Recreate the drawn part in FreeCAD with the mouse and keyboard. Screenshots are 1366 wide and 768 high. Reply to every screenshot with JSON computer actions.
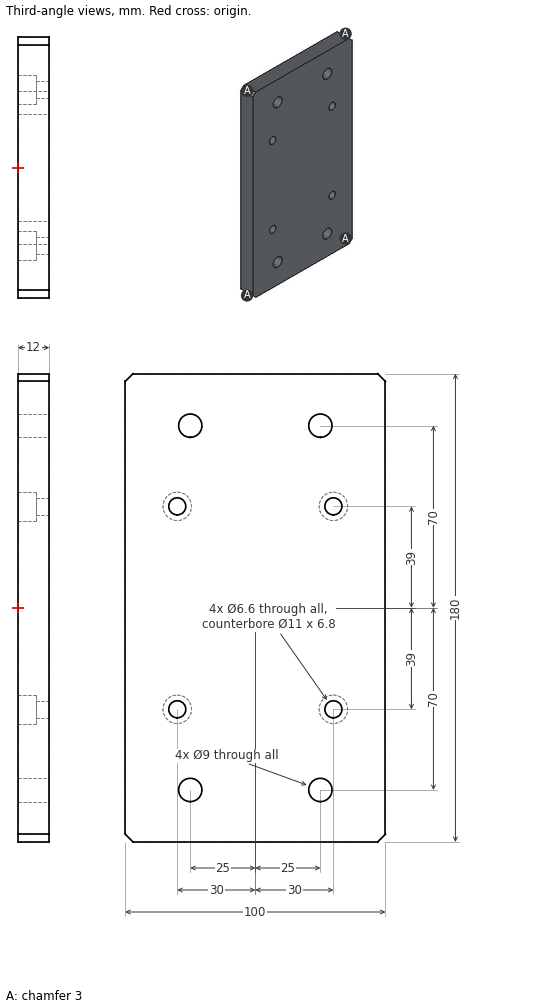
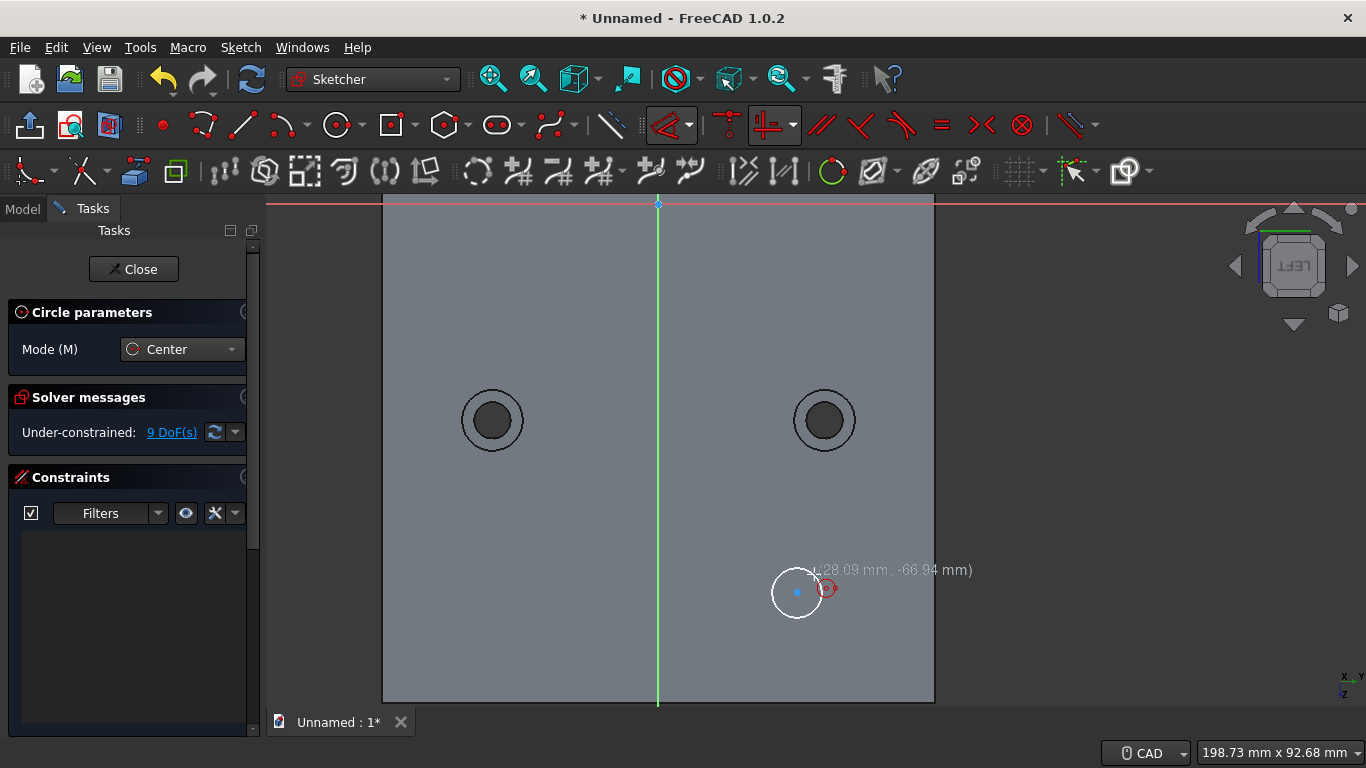
{"action": "left_click", "coordinate": [520, 592]}
{"action": "left_click", "coordinate": [538, 574]}
{"action": "key", "text": "Escape"}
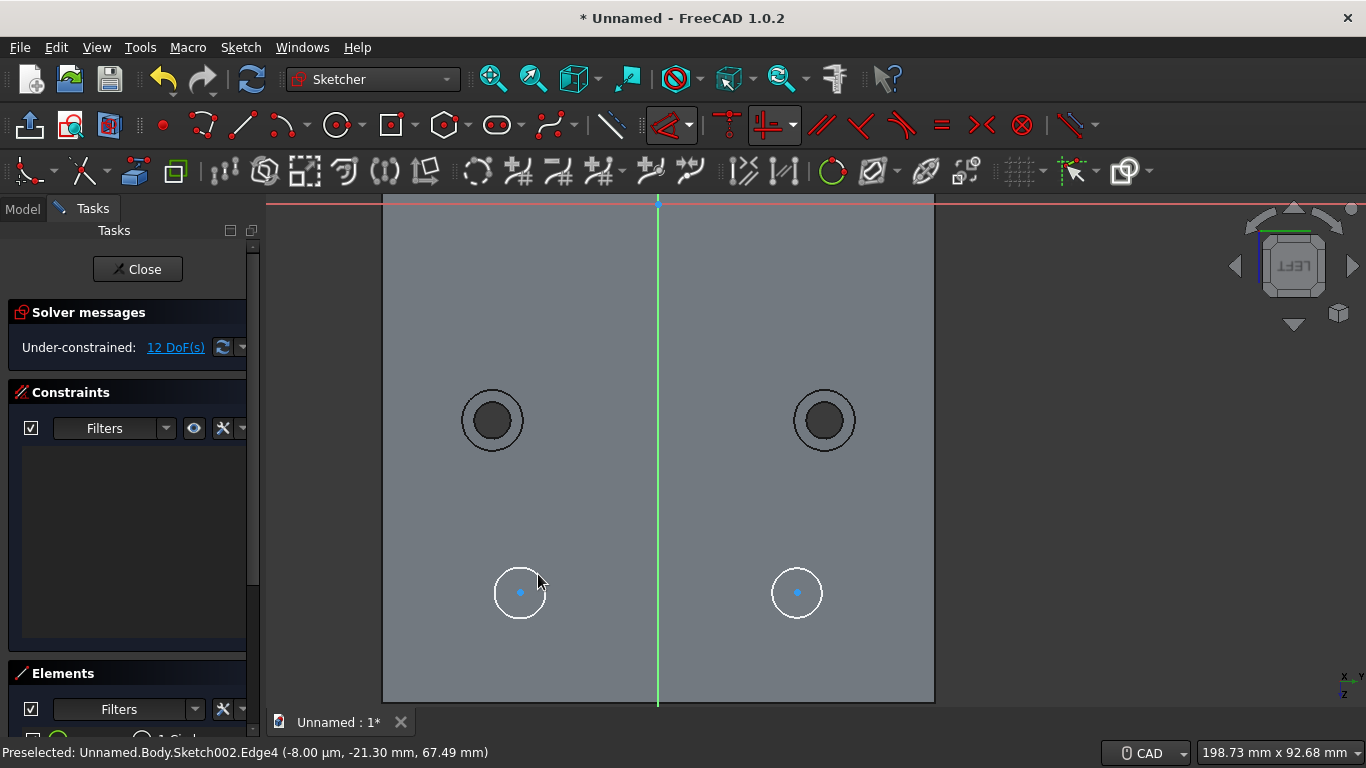
{"action": "scroll", "coordinate": [799, 594], "scroll_direction": "down", "scroll_amount": 5}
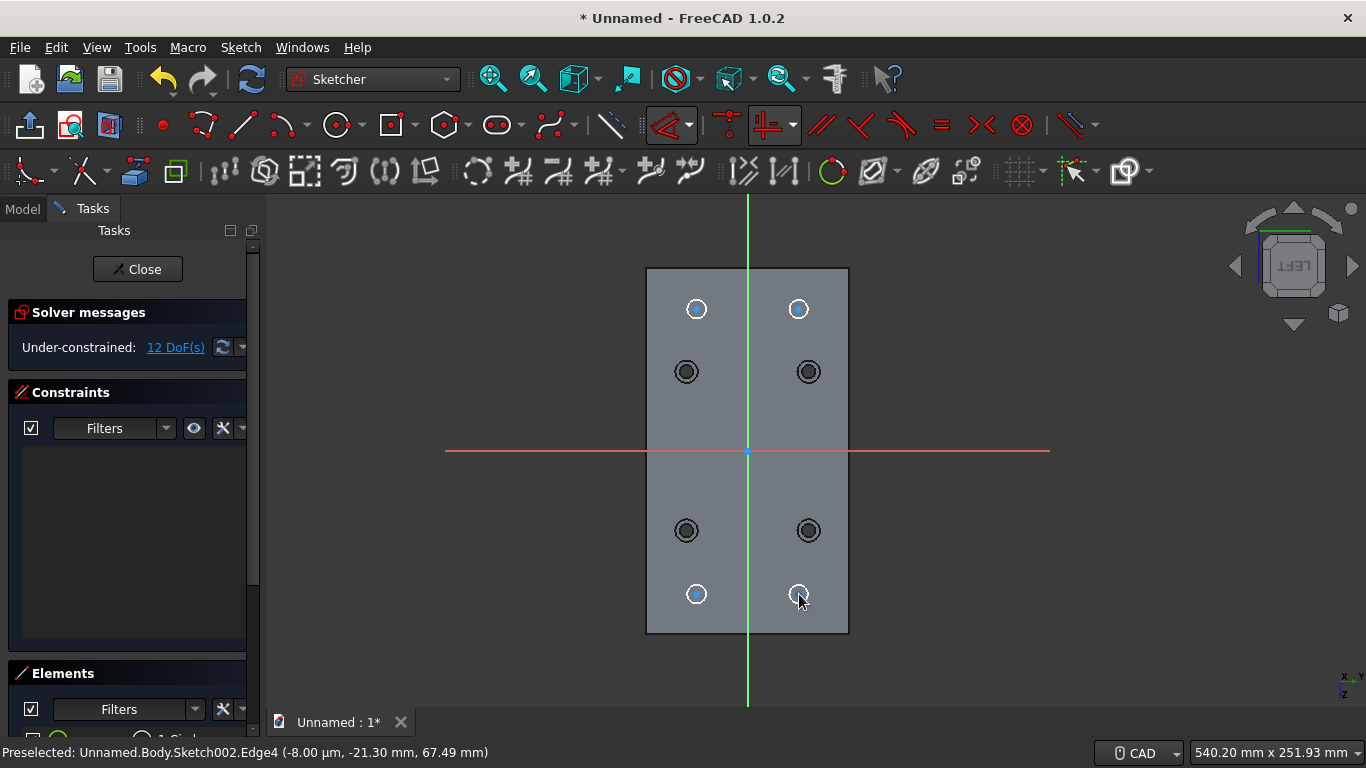
{"action": "scroll", "coordinate": [805, 303], "scroll_direction": "up", "scroll_amount": 3}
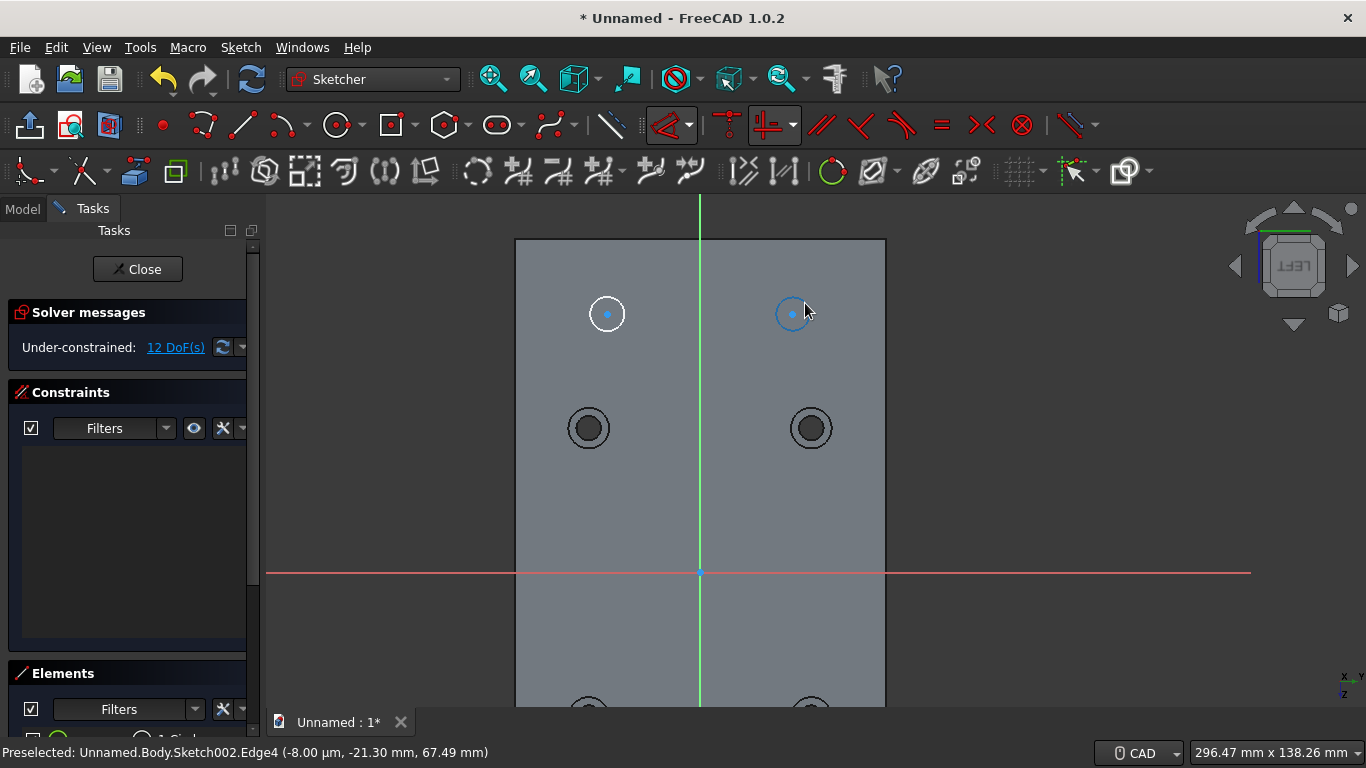
{"action": "left_click", "coordinate": [805, 302]}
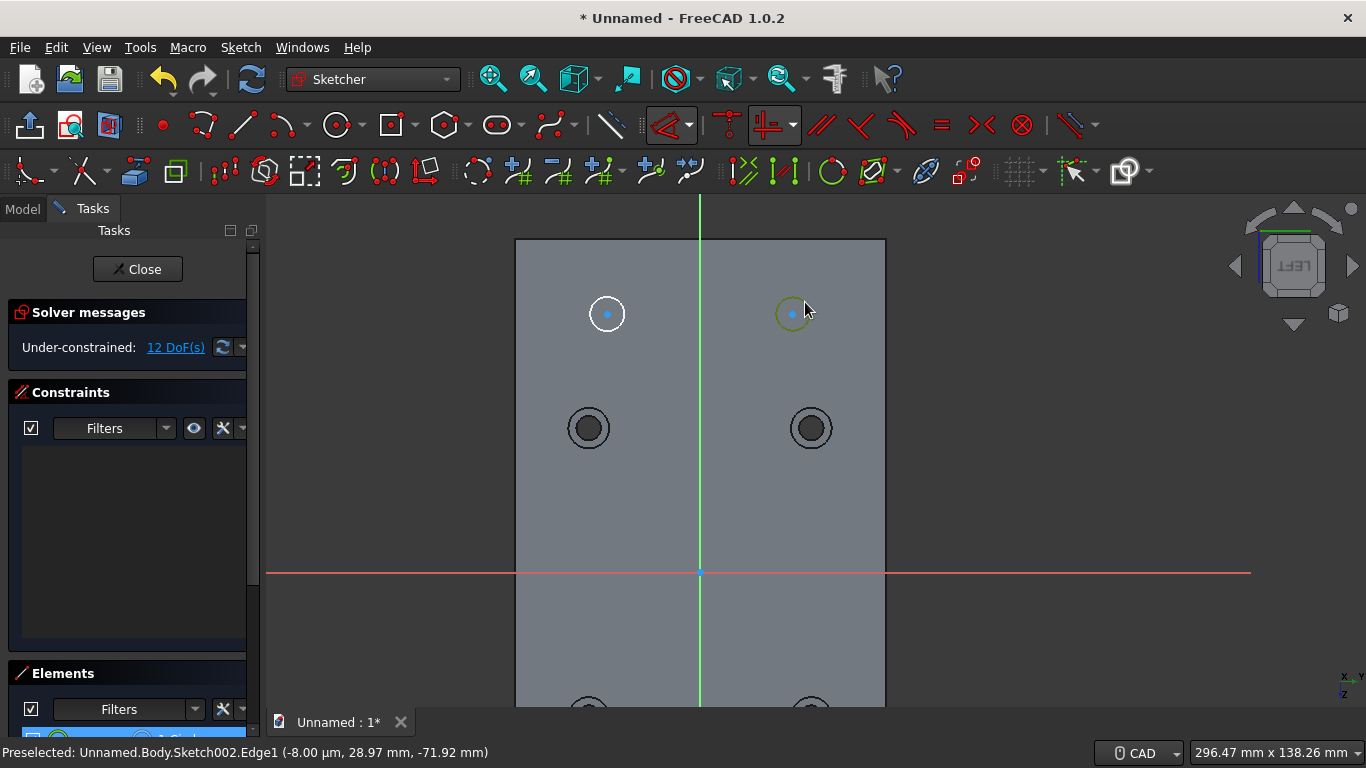
{"action": "left_click", "coordinate": [619, 302]}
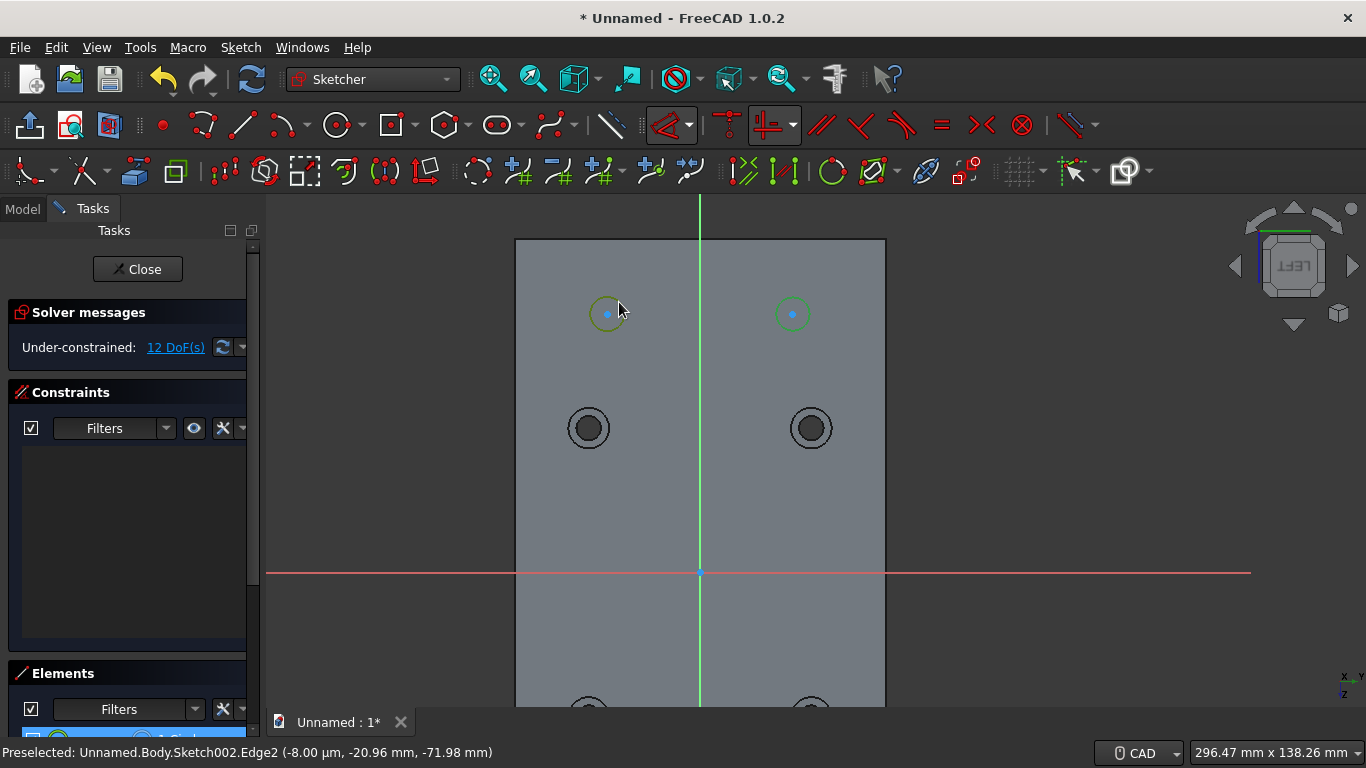
{"action": "scroll", "coordinate": [805, 302], "scroll_direction": "down", "scroll_amount": 3}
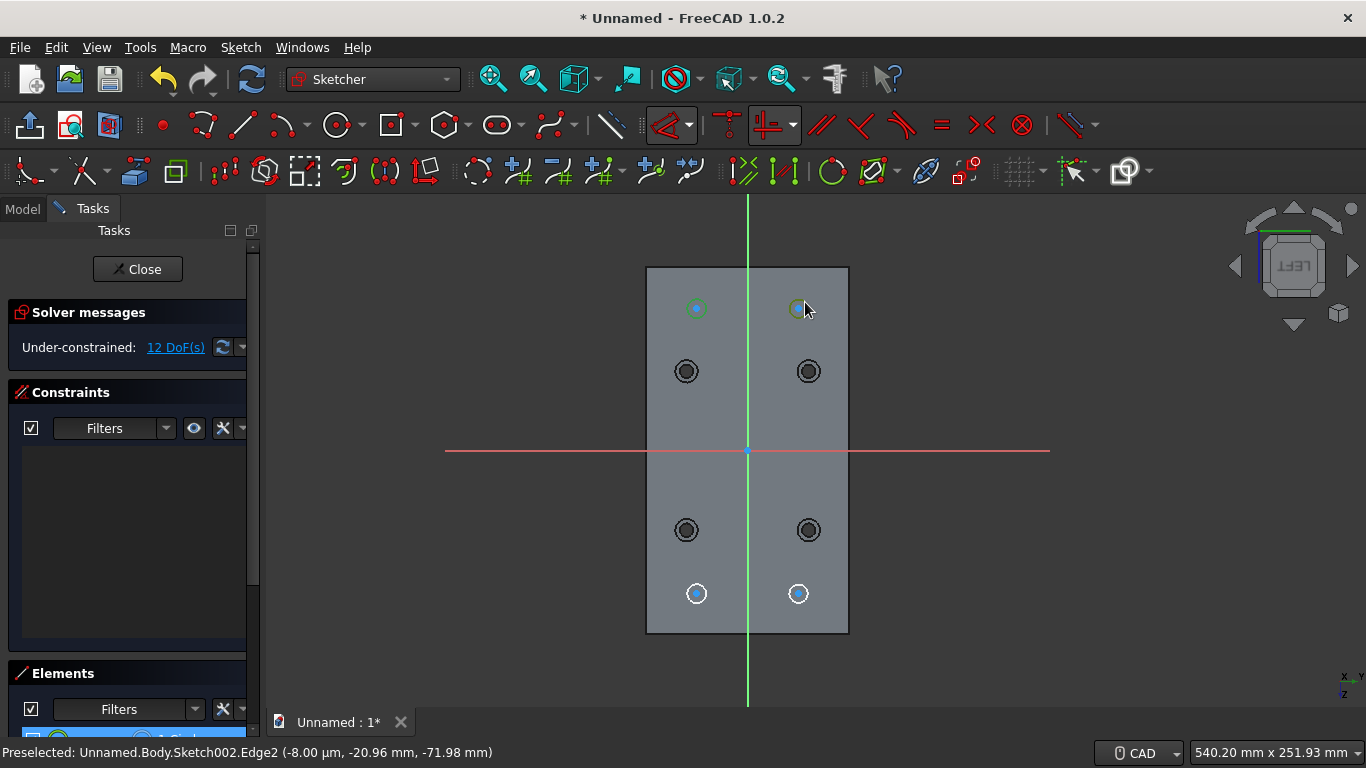
{"action": "scroll", "coordinate": [805, 587], "scroll_direction": "up", "scroll_amount": 3}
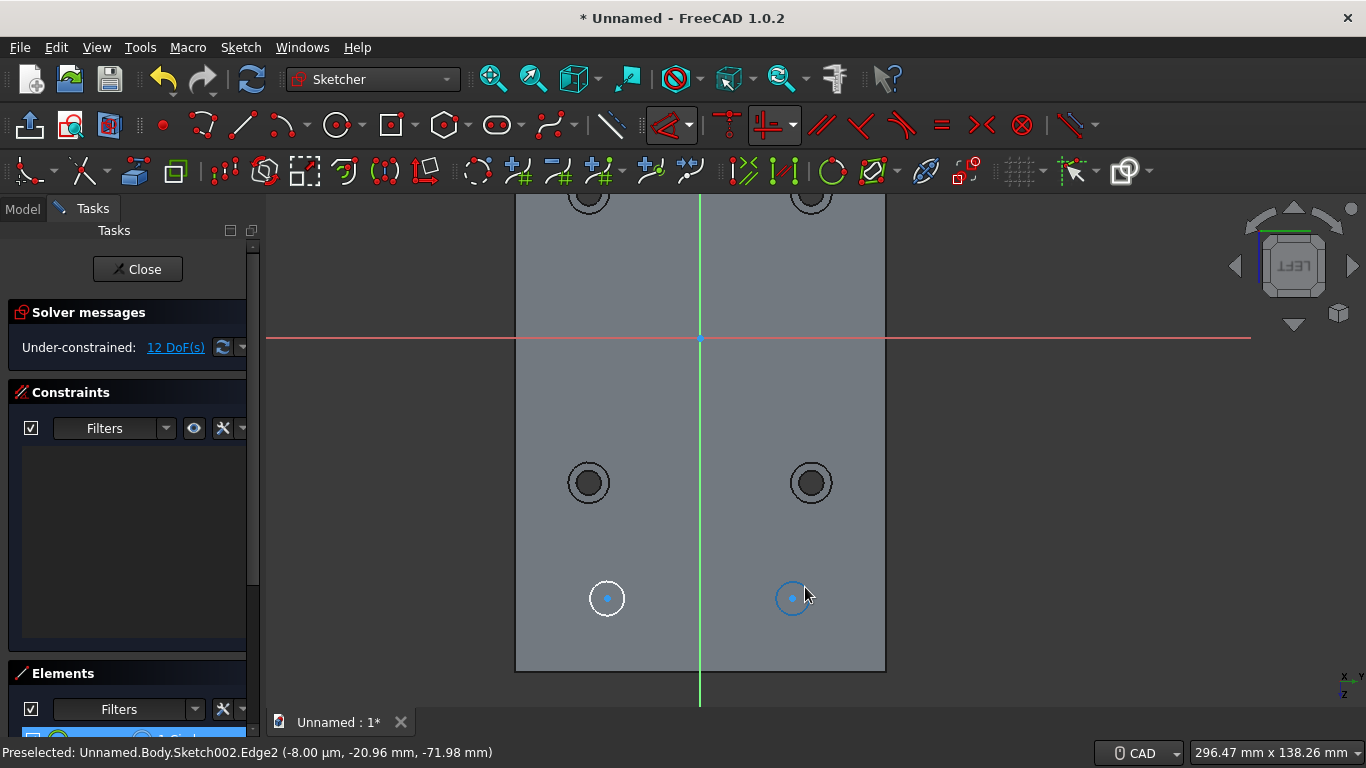
{"action": "left_click", "coordinate": [805, 587]}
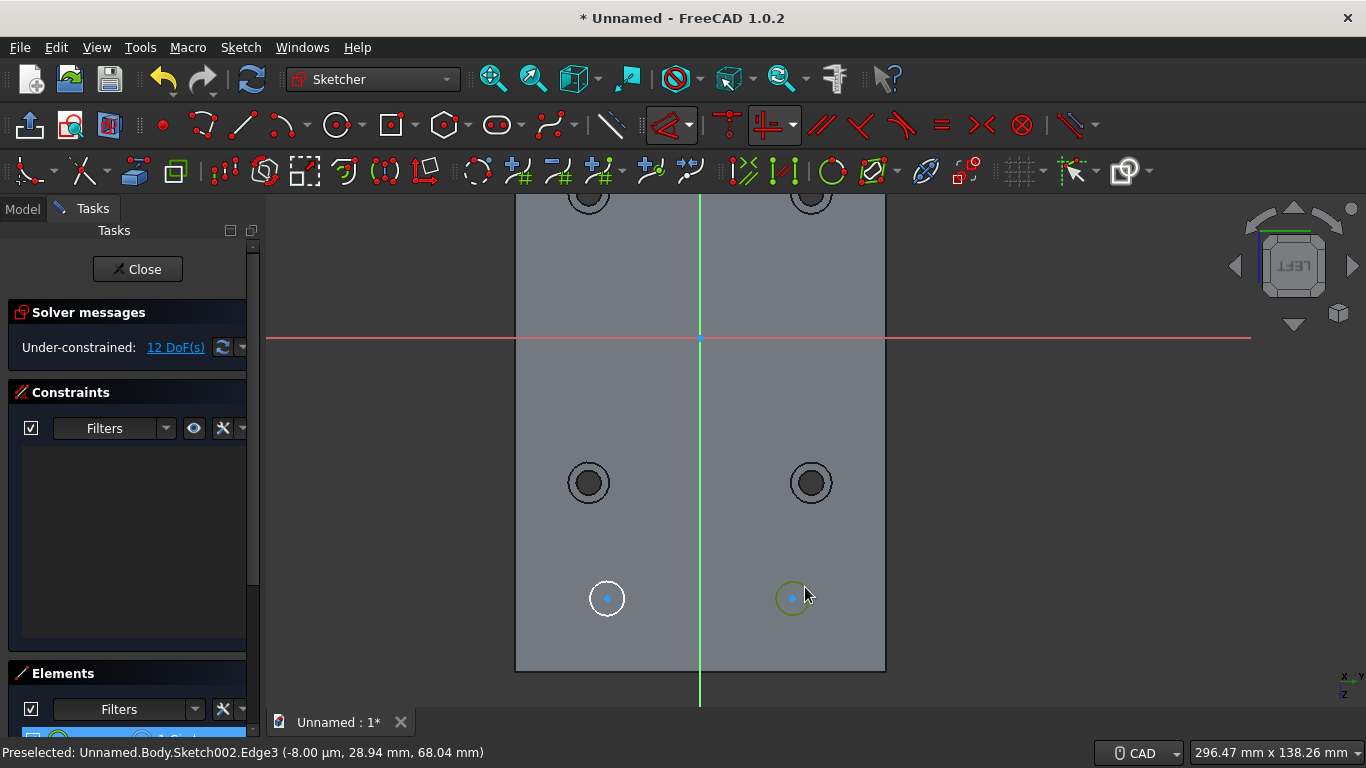
{"action": "left_click", "coordinate": [619, 586]}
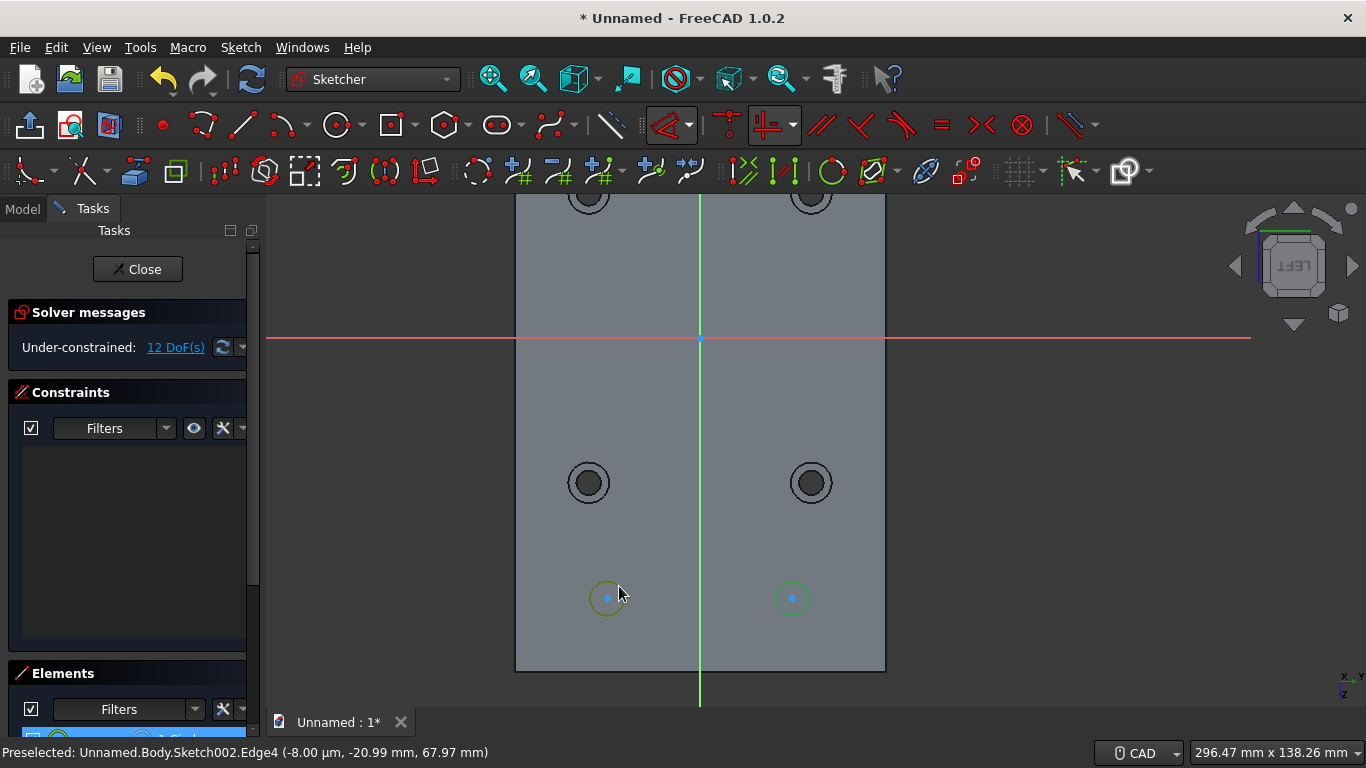
{"action": "left_click", "coordinate": [942, 126]}